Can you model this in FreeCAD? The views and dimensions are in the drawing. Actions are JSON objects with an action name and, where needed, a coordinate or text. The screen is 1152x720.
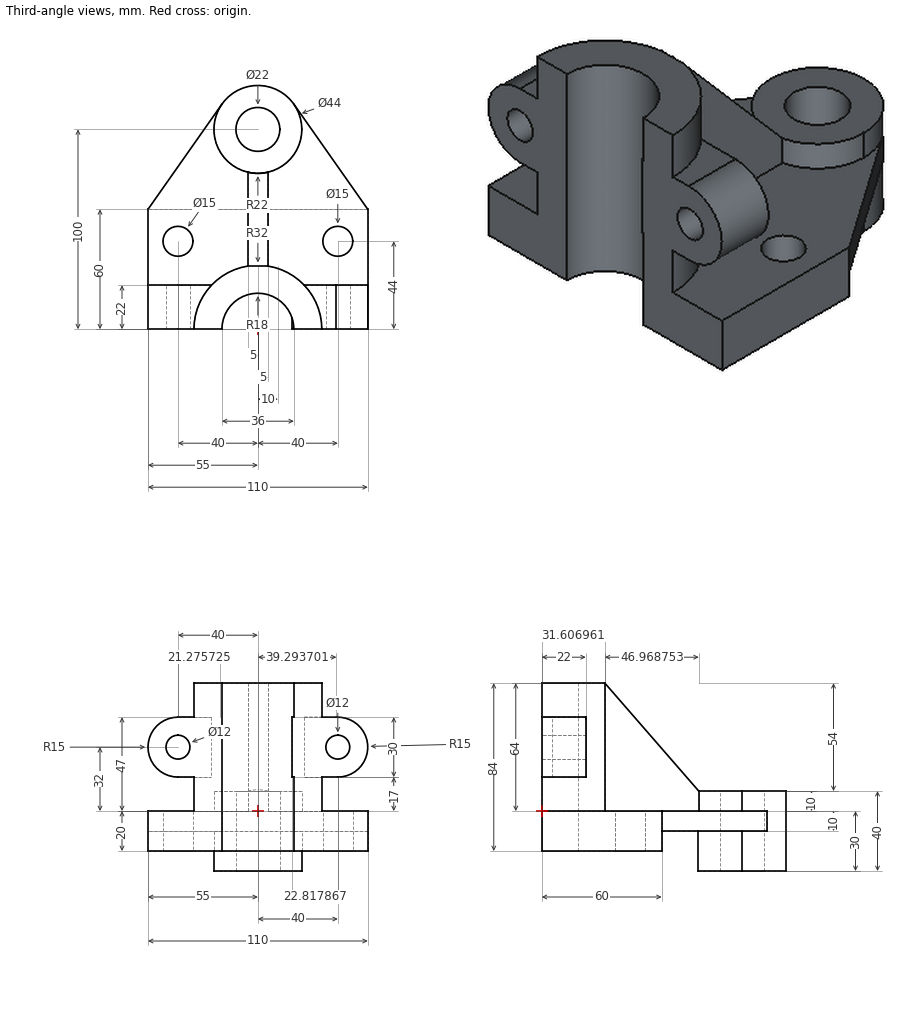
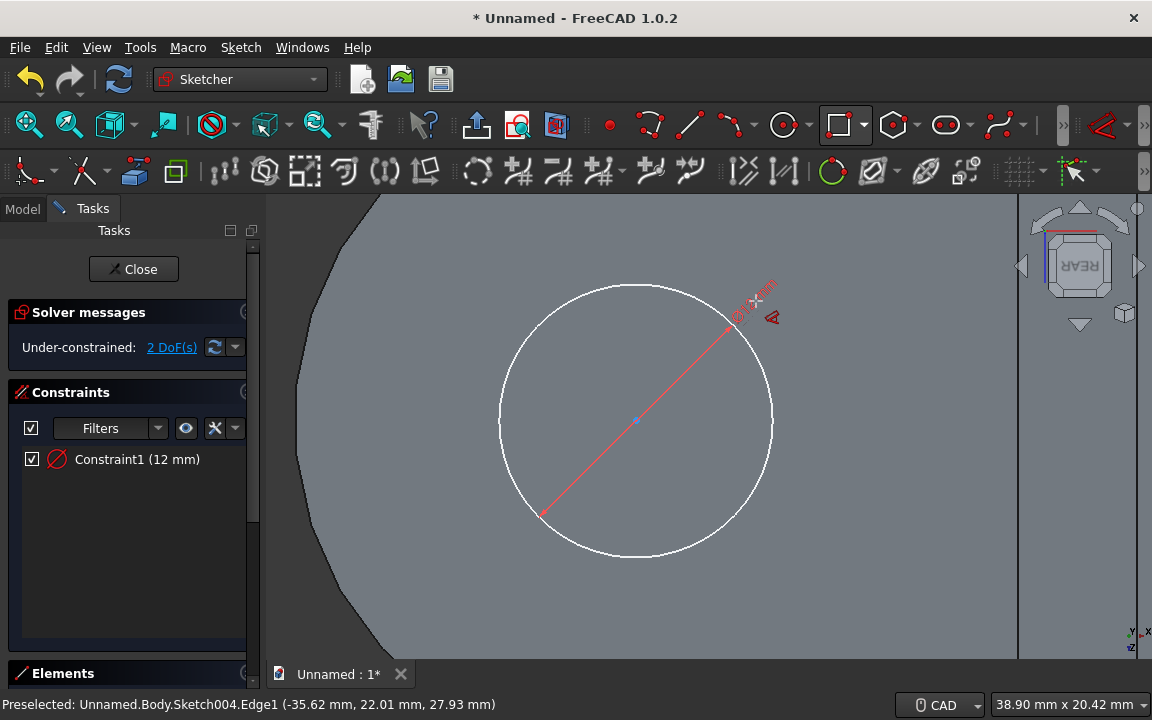
{"action": "left_click", "coordinate": [636, 421]}
{"action": "left_click", "coordinate": [811, 455]}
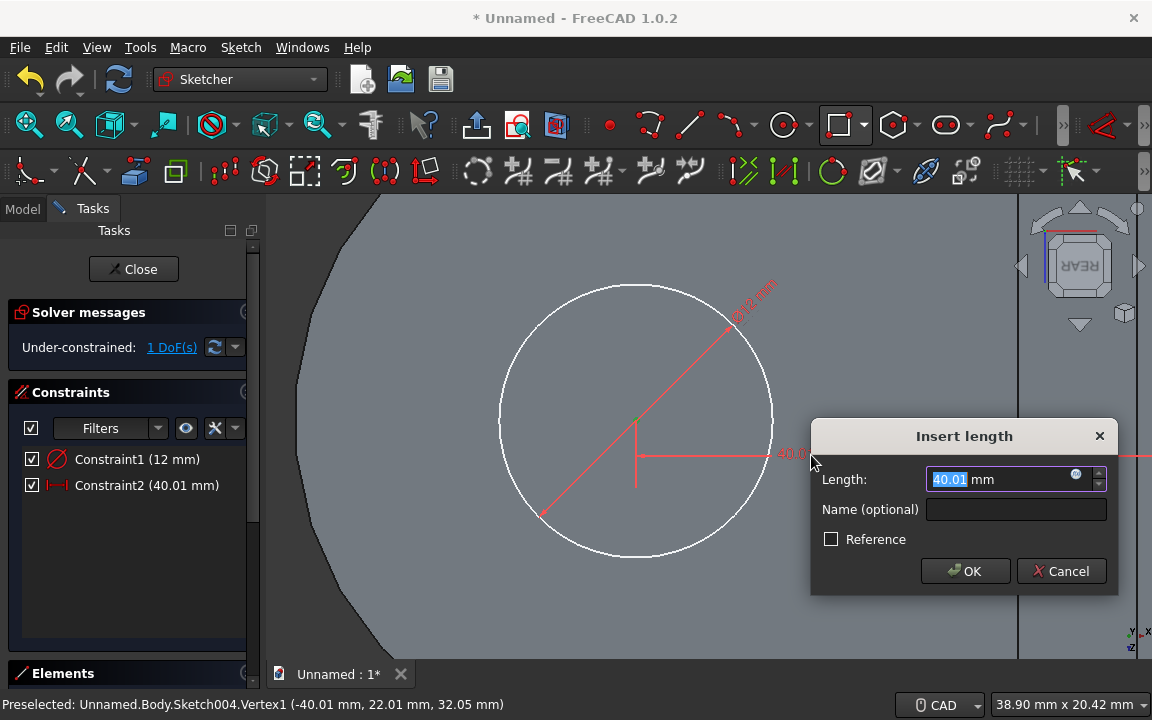
{"action": "type", "text": "40"}
{"action": "key", "text": "Return"}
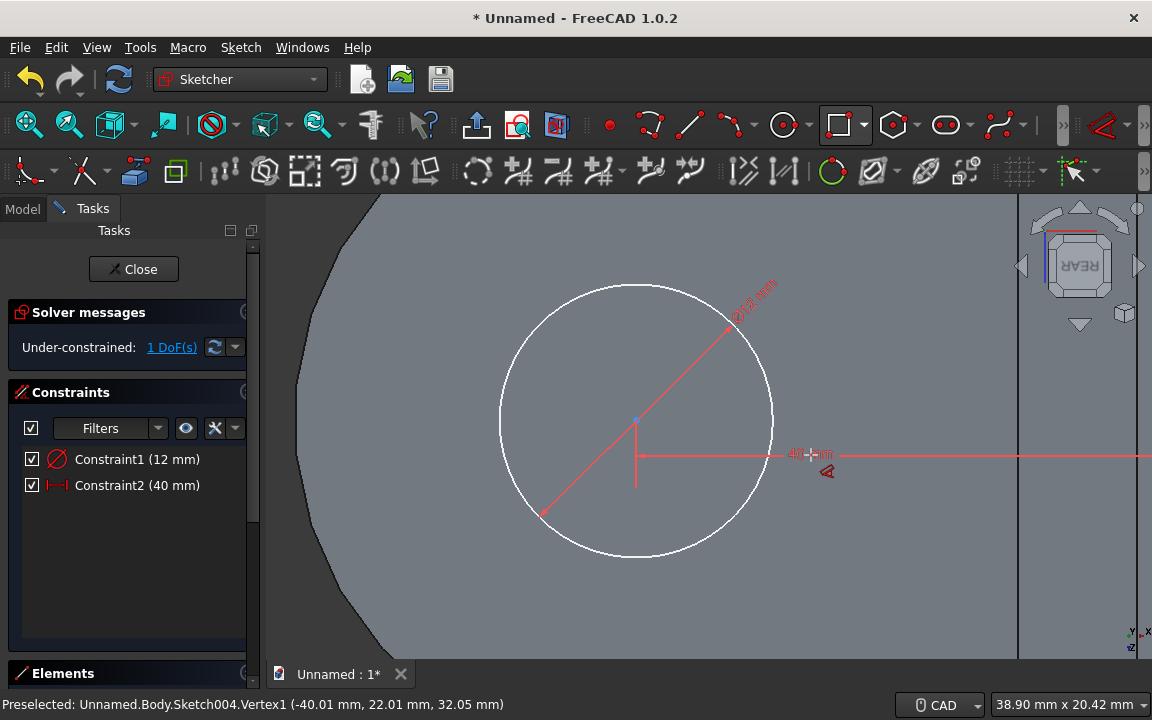
{"action": "left_click", "coordinate": [636, 421]}
{"action": "left_click", "coordinate": [602, 321]}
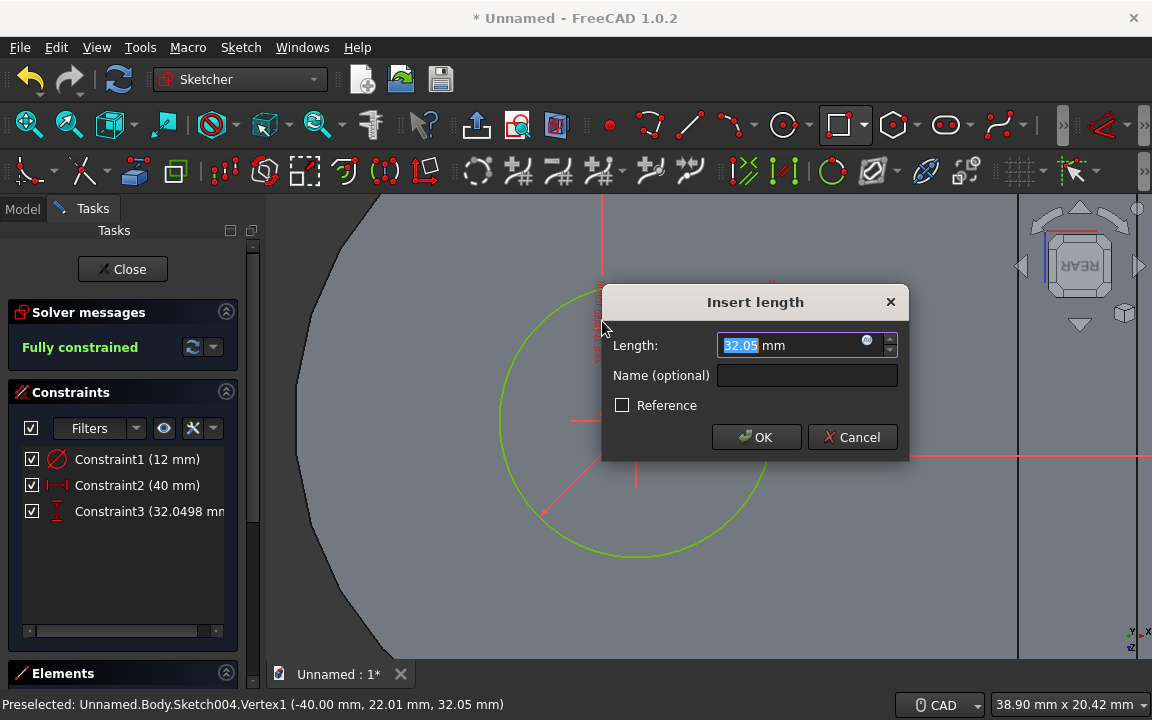
{"action": "type", "text": "32"}
{"action": "key", "text": "Return"}
{"action": "key", "text": "Escape"}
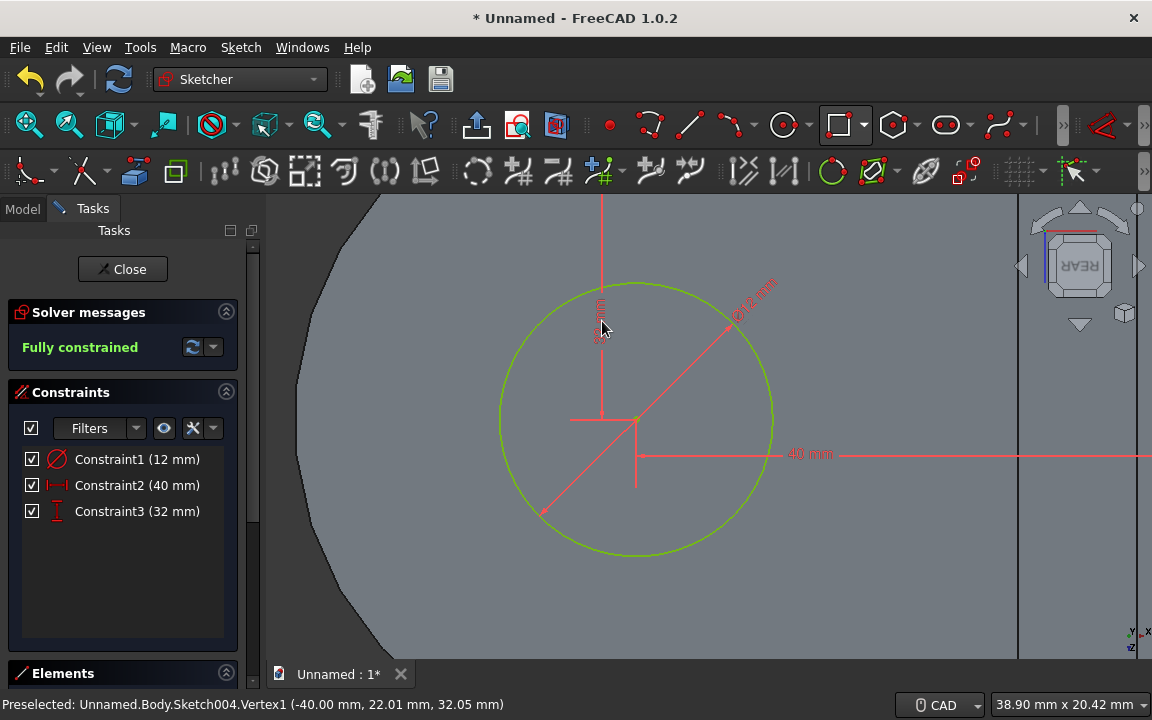
{"action": "left_click", "coordinate": [123, 269]}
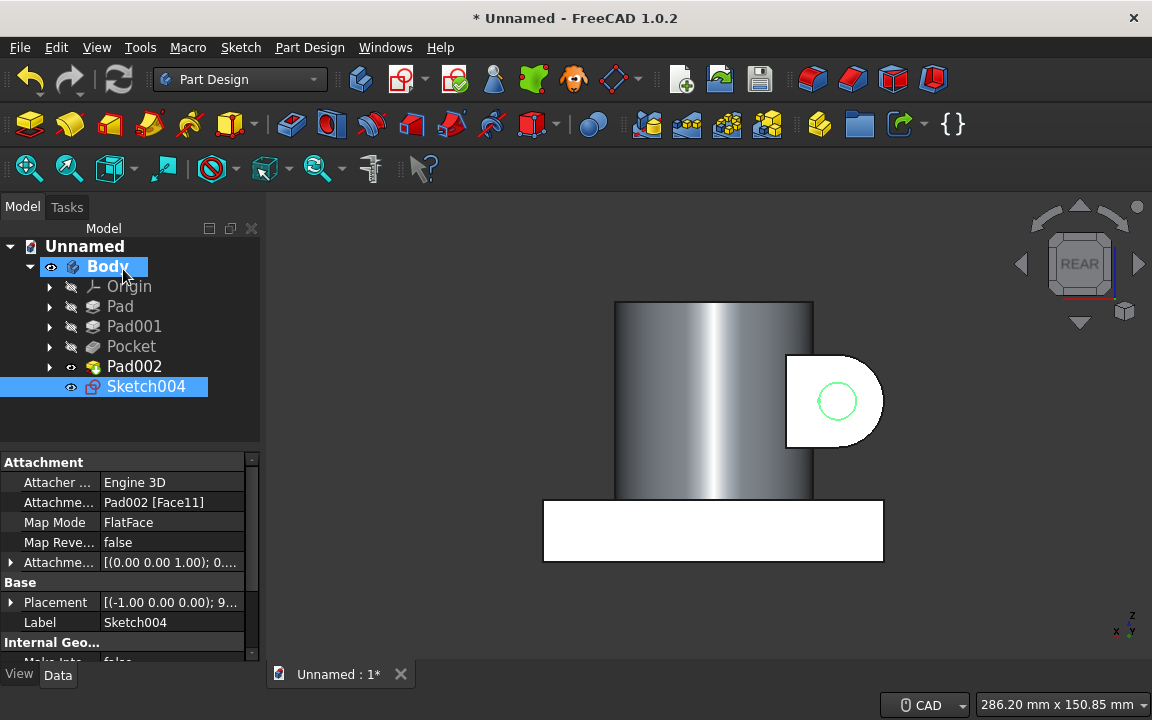
{"action": "left_click", "coordinate": [292, 124]}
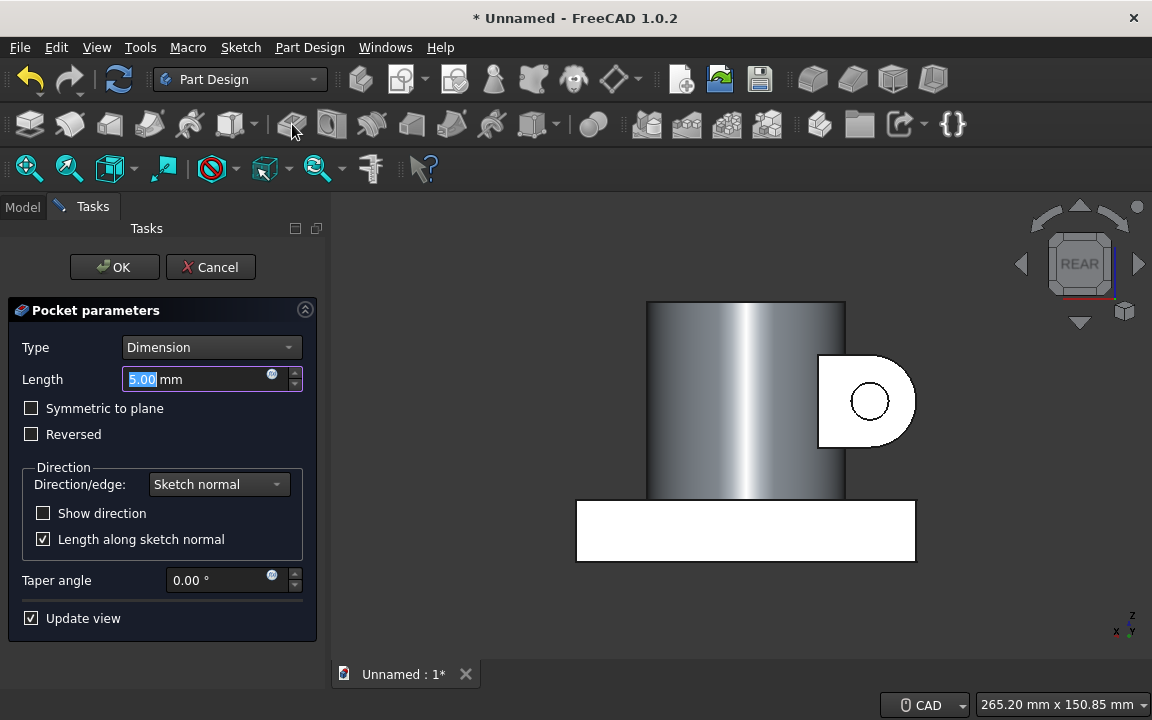
{"action": "type", "text": "22"}
{"action": "key", "text": "Tab"}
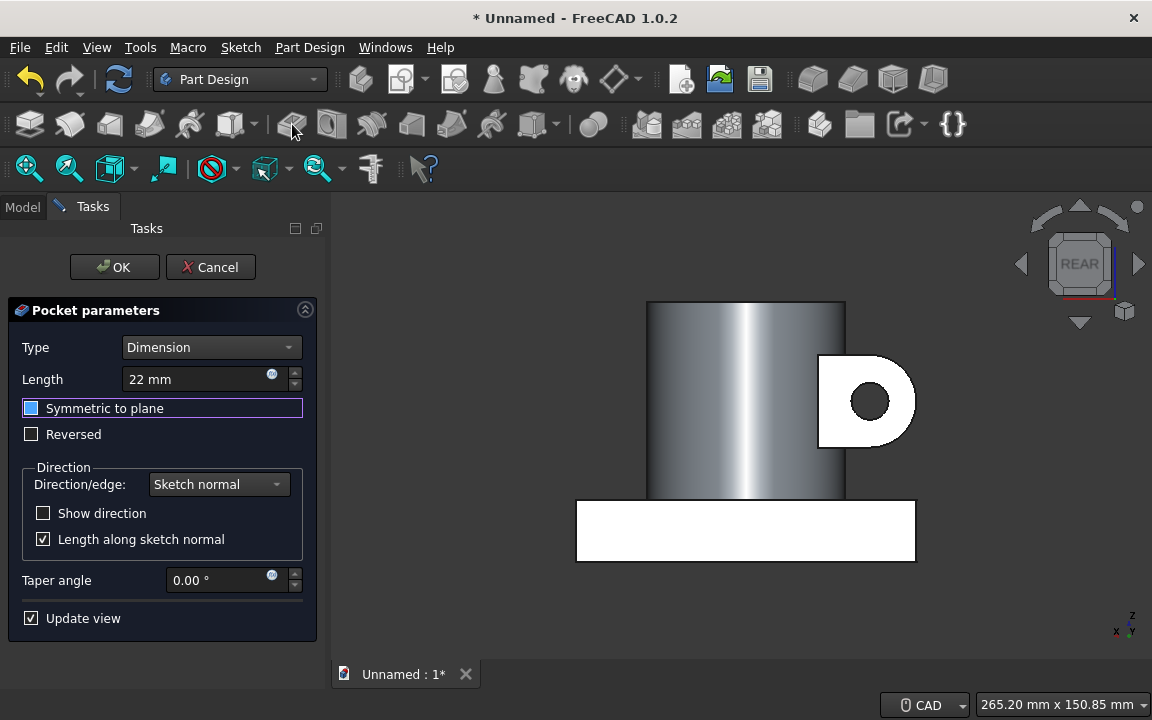
{"action": "left_click", "coordinate": [115, 267]}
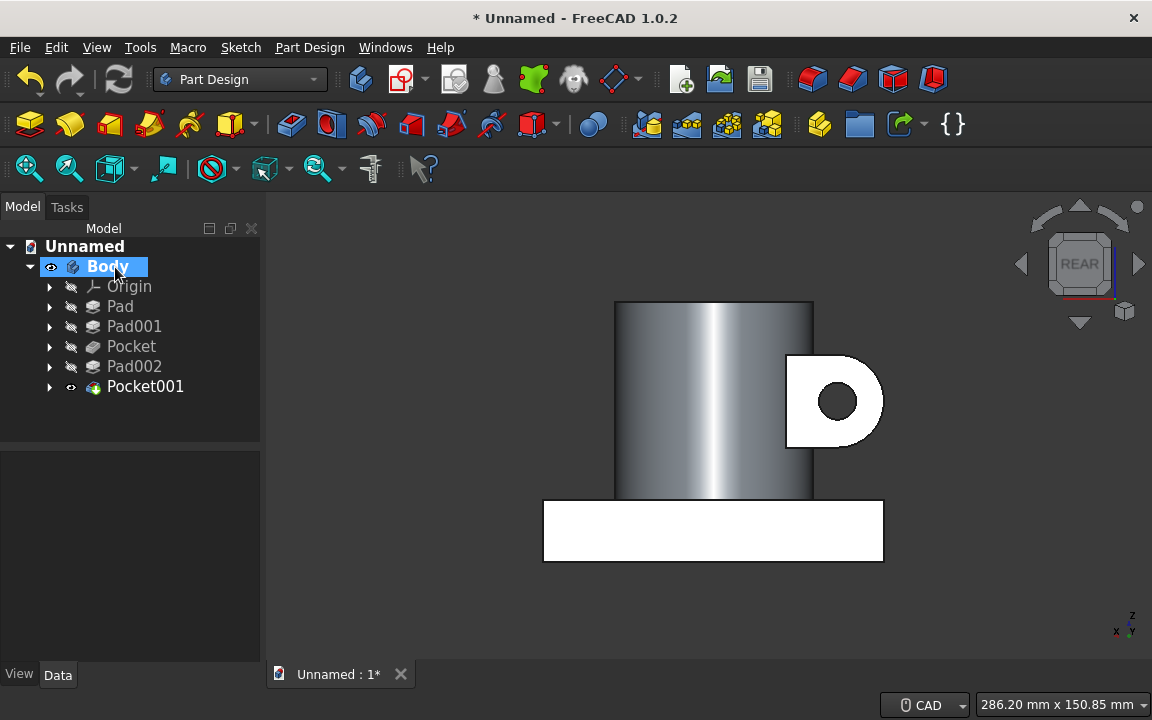
{"action": "left_click", "coordinate": [402, 80]}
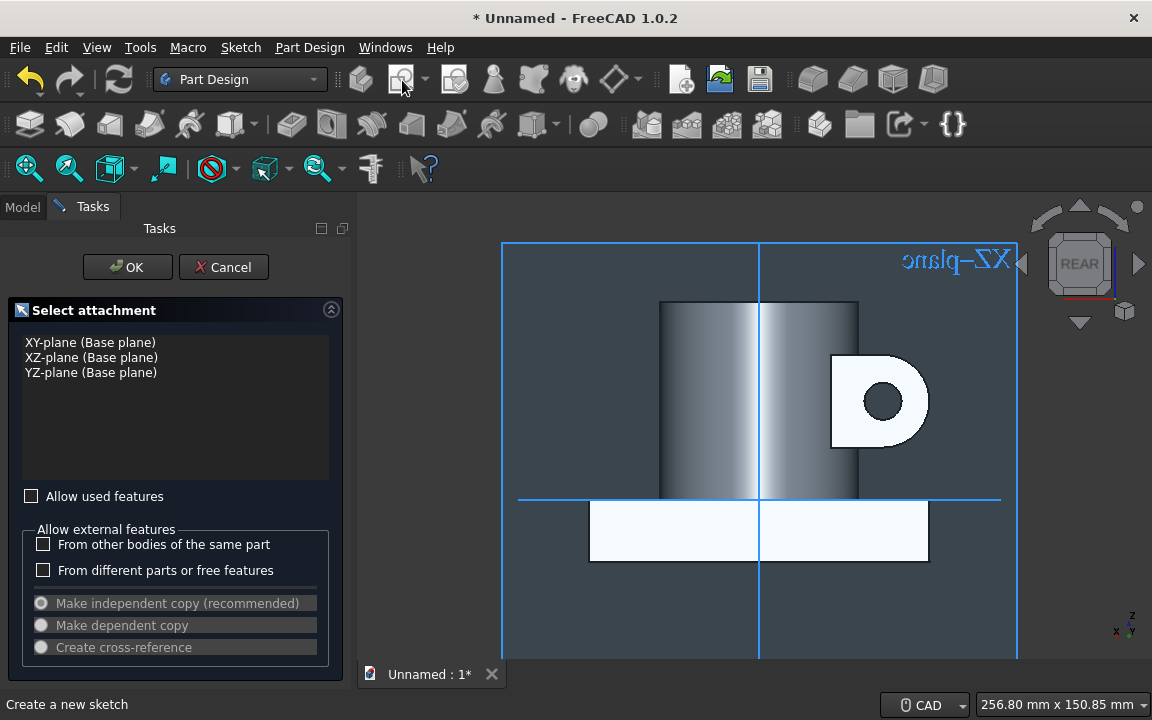
{"action": "left_click", "coordinate": [82, 358]}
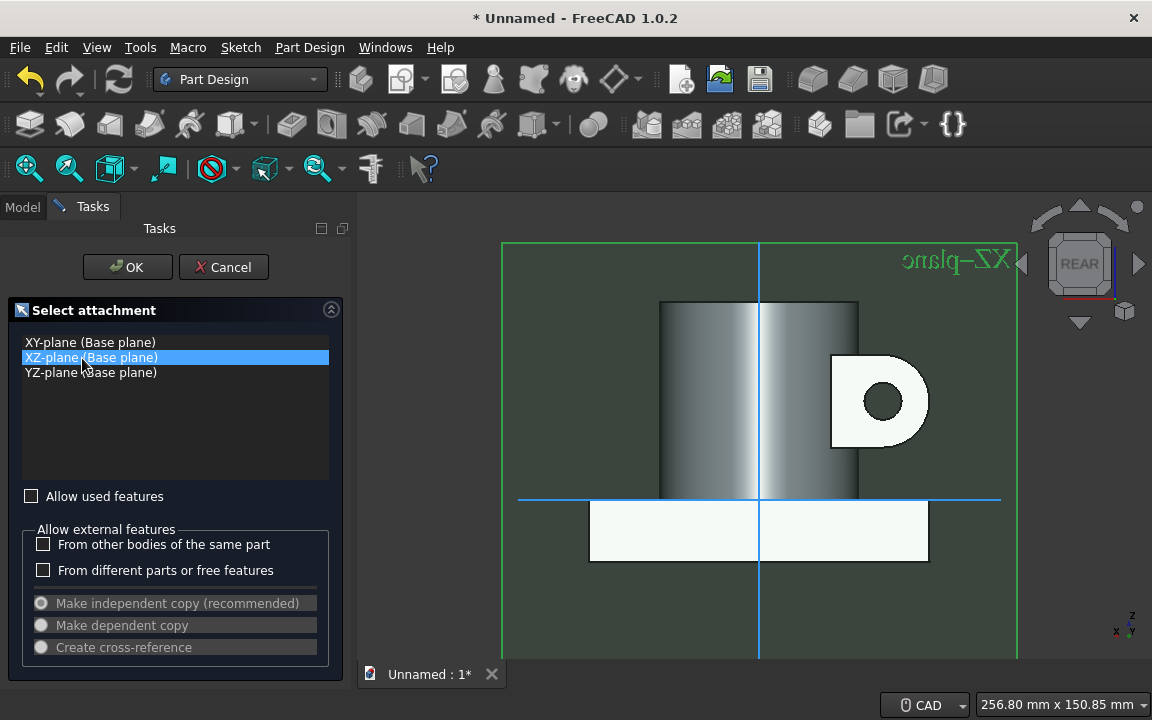
{"action": "left_click", "coordinate": [128, 267]}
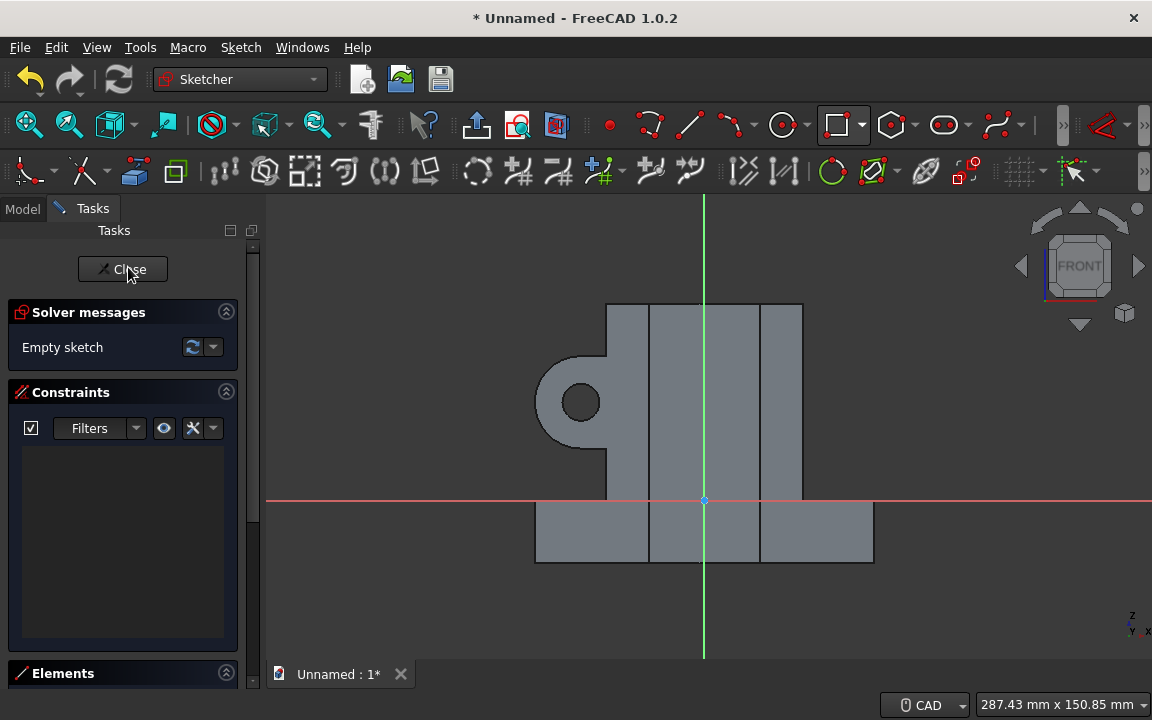
{"action": "scroll", "coordinate": [970, 431], "scroll_direction": "up", "scroll_amount": 3}